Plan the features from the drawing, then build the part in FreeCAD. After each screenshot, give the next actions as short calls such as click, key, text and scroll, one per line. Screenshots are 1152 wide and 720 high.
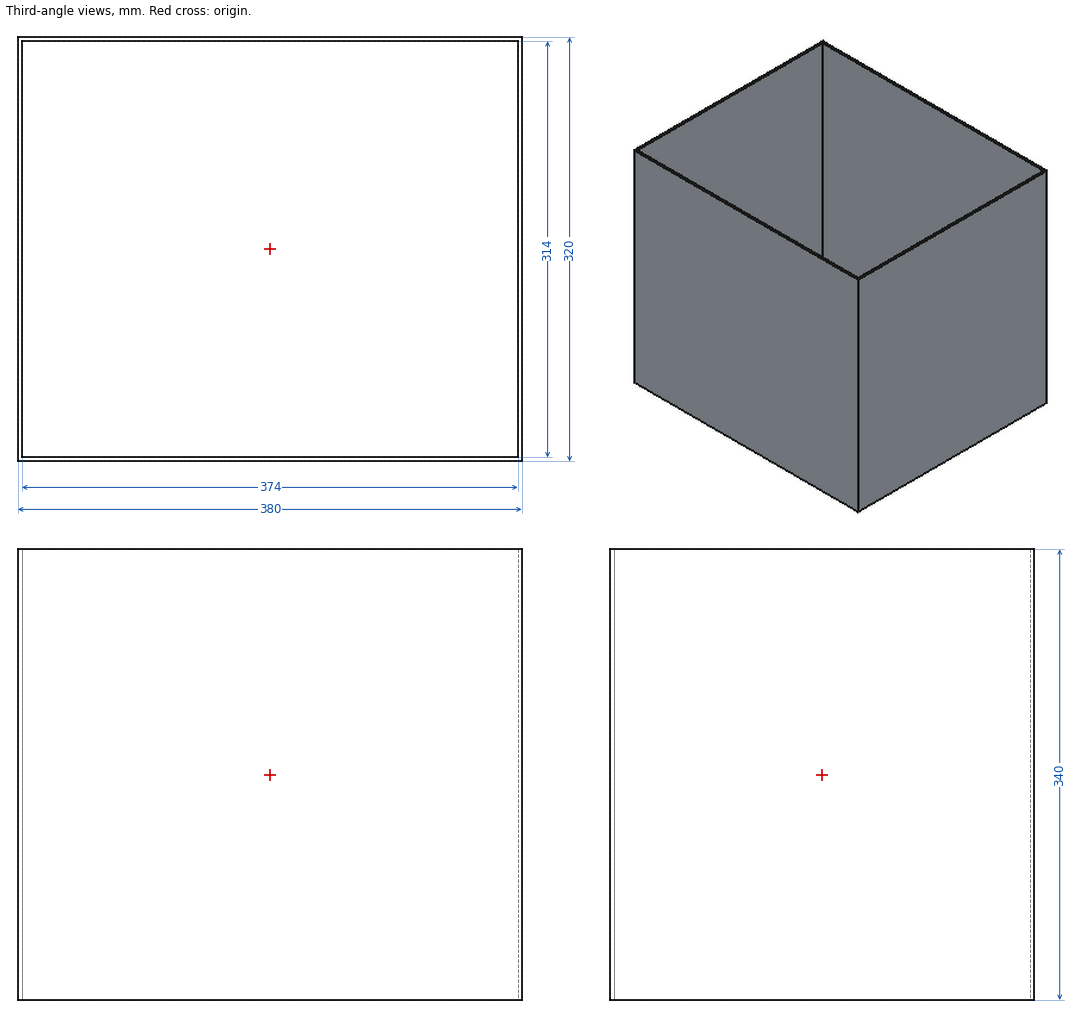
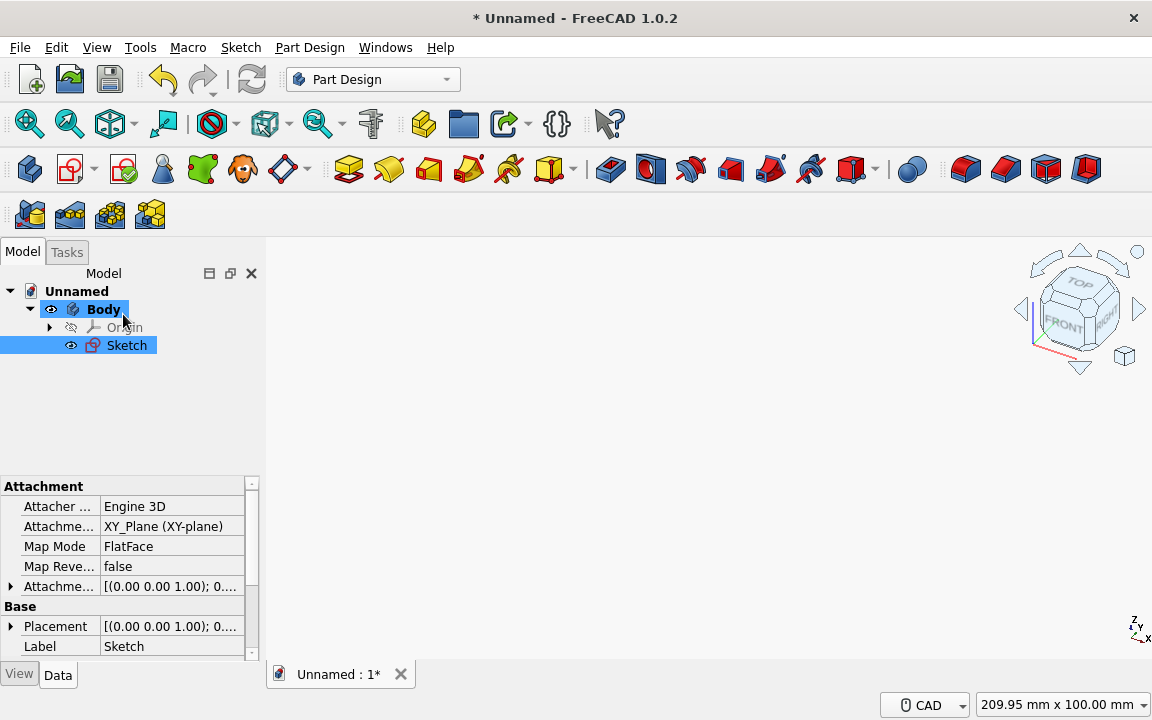
click(350, 170)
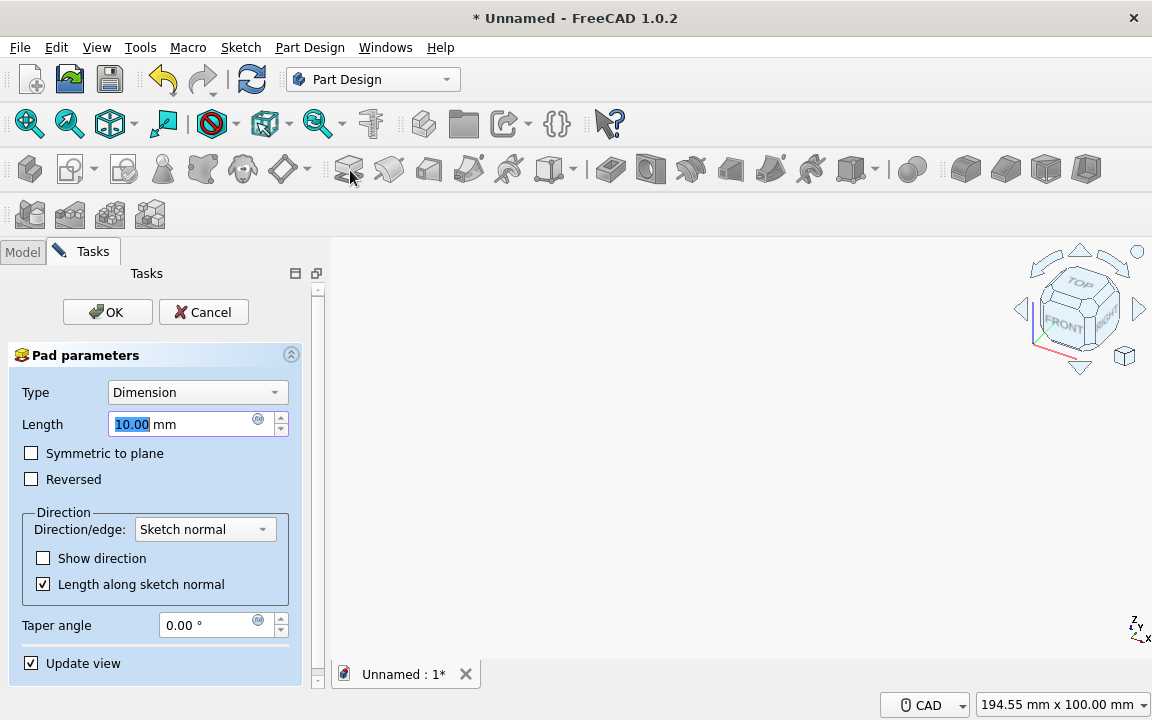
text(340)
key(Tab)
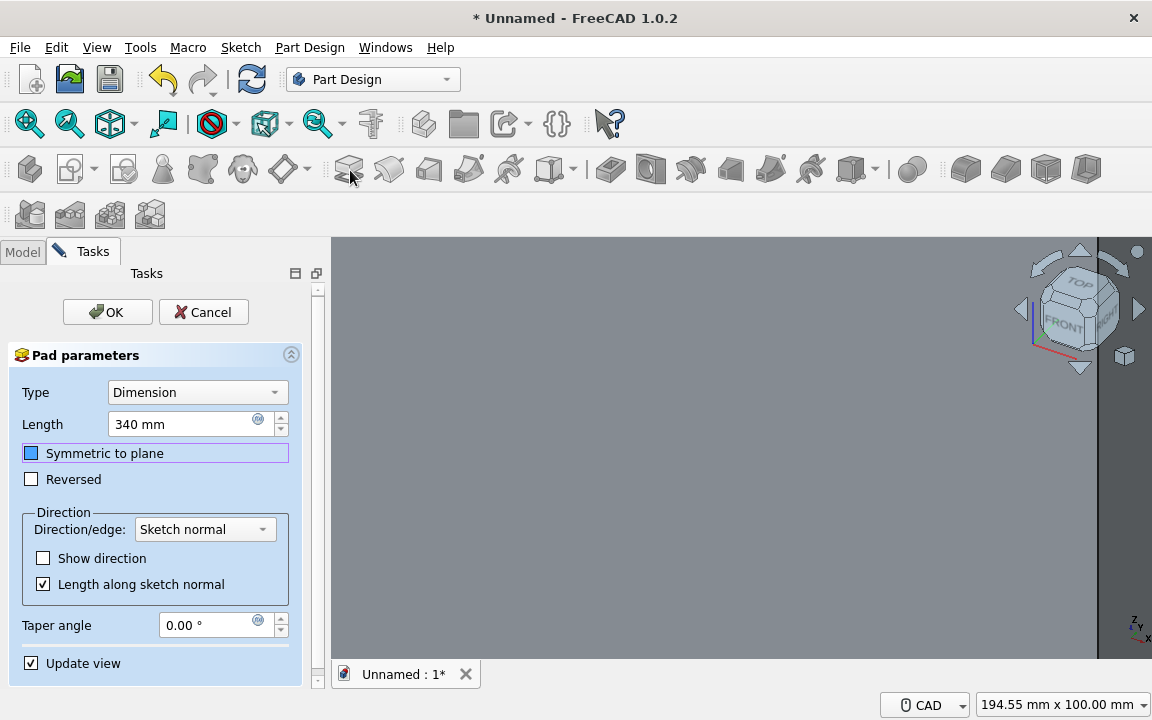
click(30, 453)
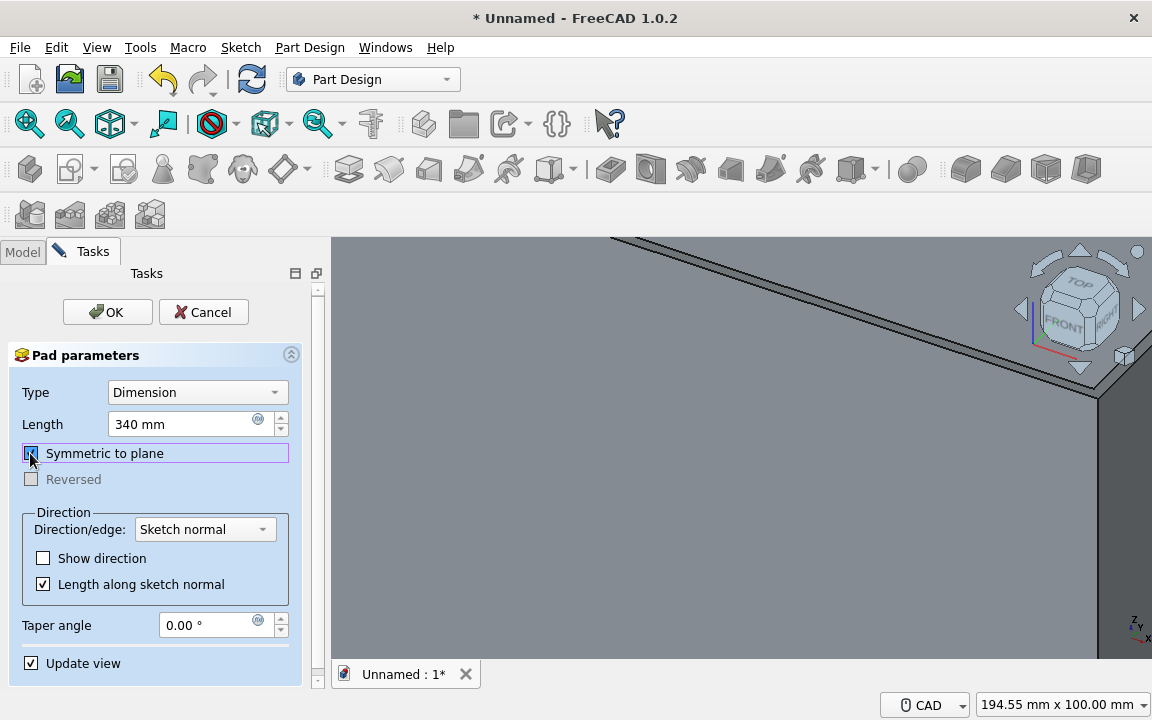
click(108, 312)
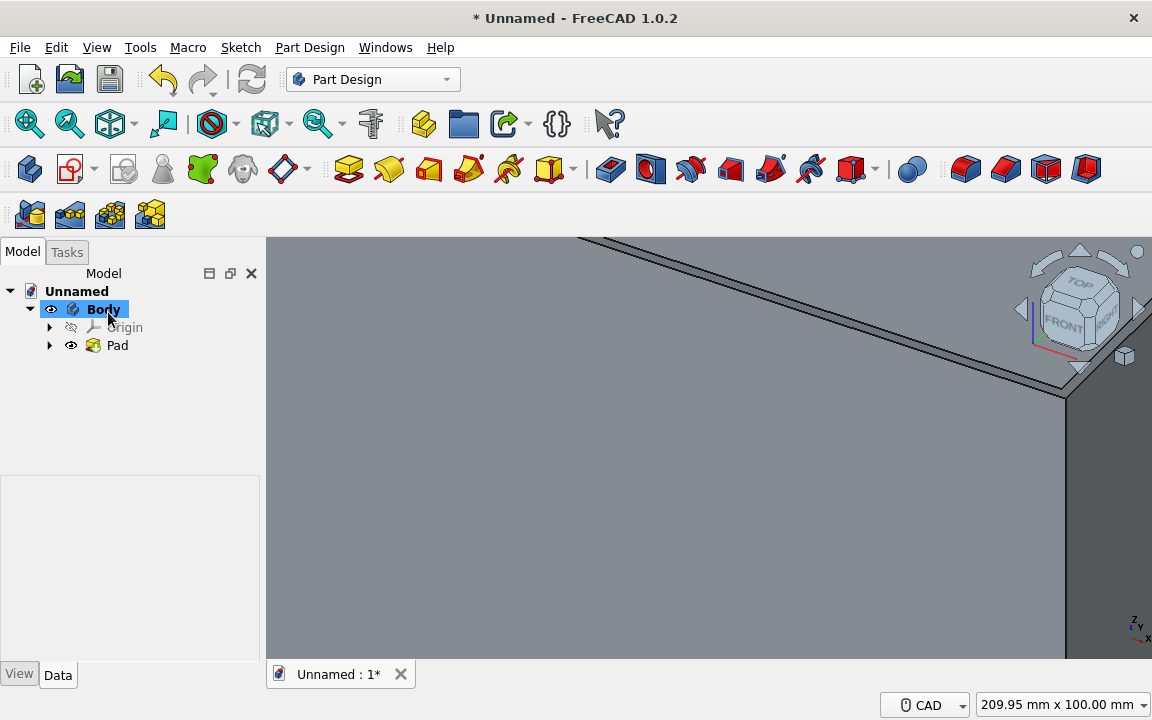
key(0)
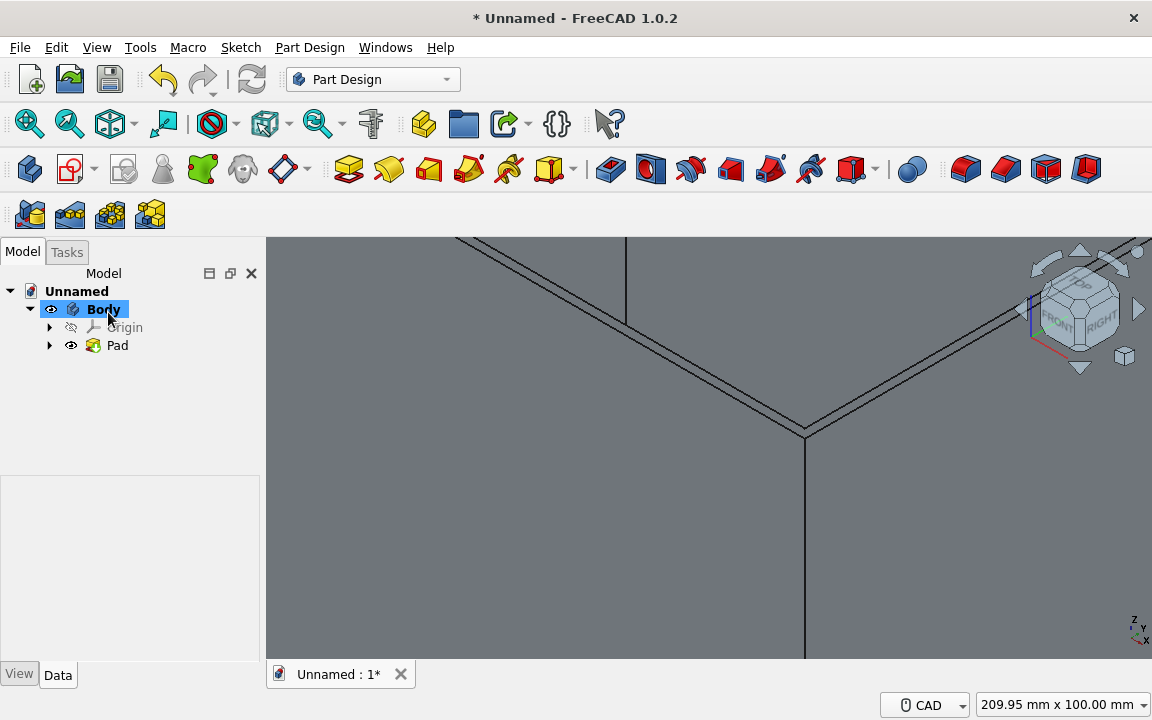
click(30, 124)